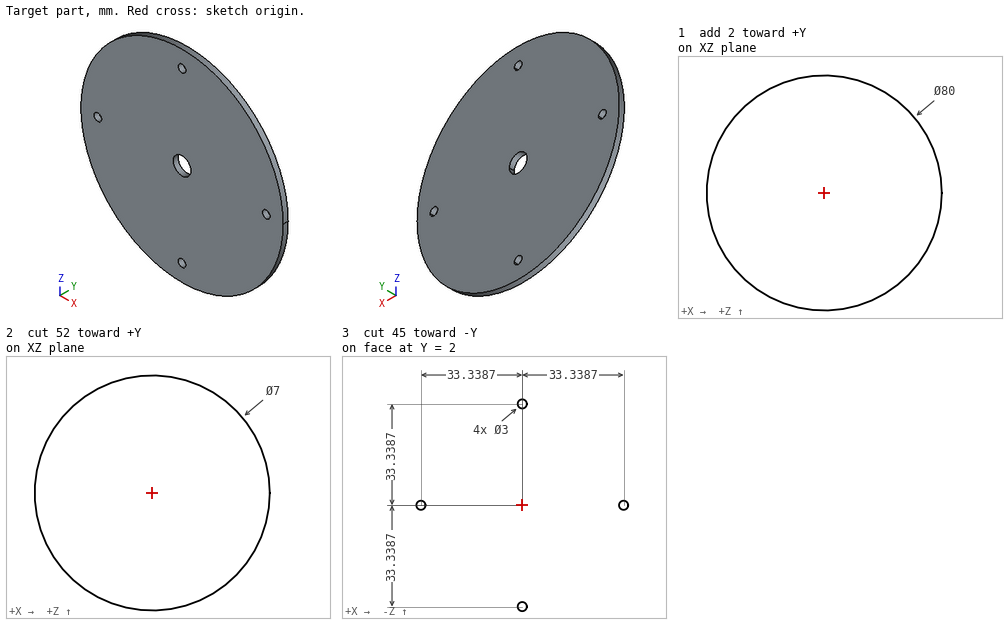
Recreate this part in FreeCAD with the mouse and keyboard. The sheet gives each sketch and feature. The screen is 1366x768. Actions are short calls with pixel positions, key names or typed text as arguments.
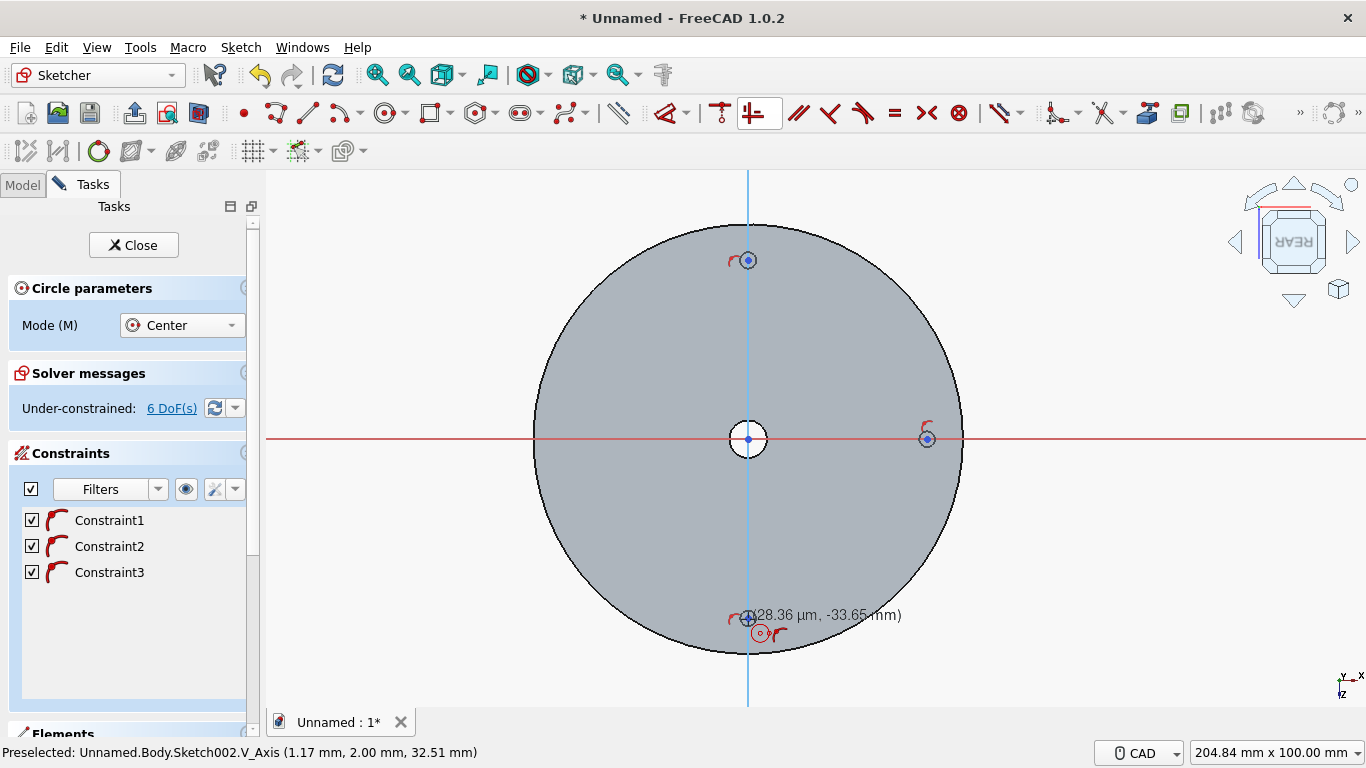
scroll(569, 439, up, 6)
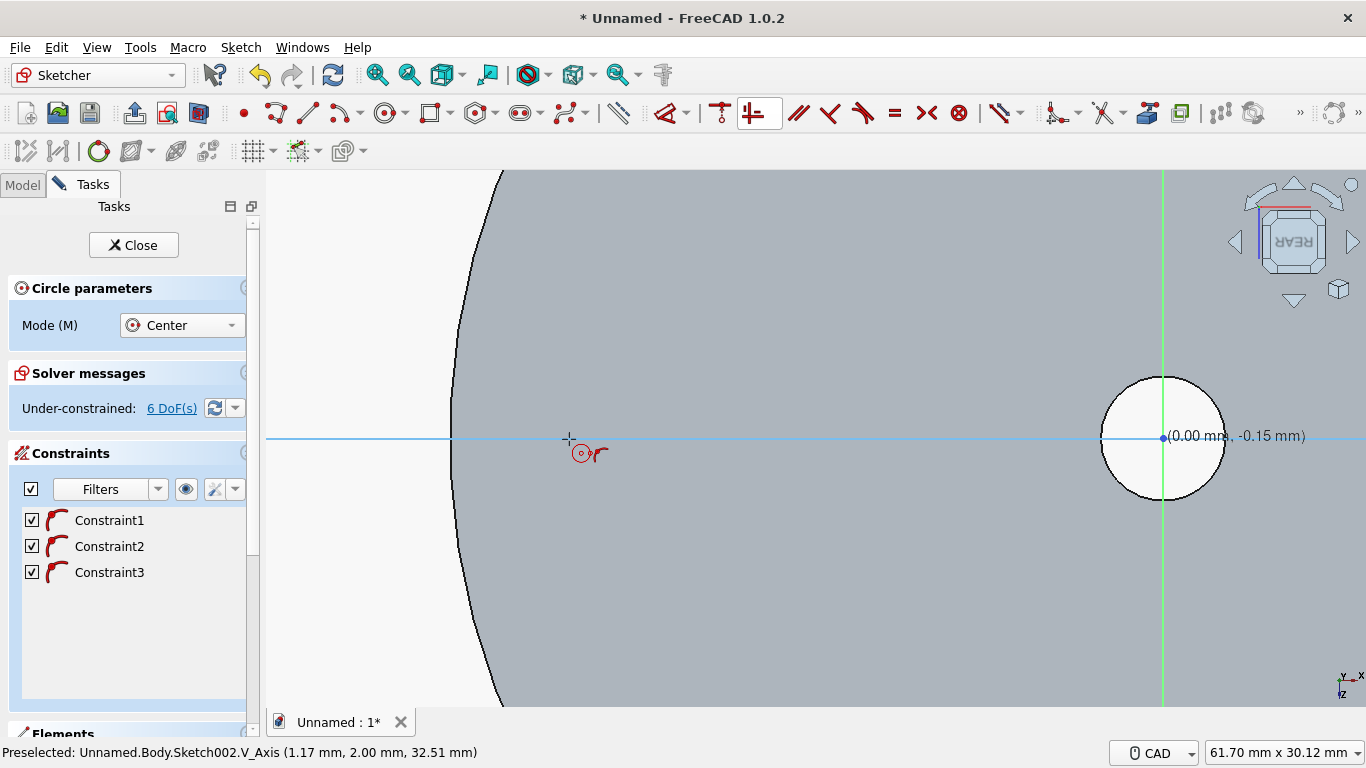
click(569, 439)
click(588, 420)
key(Escape)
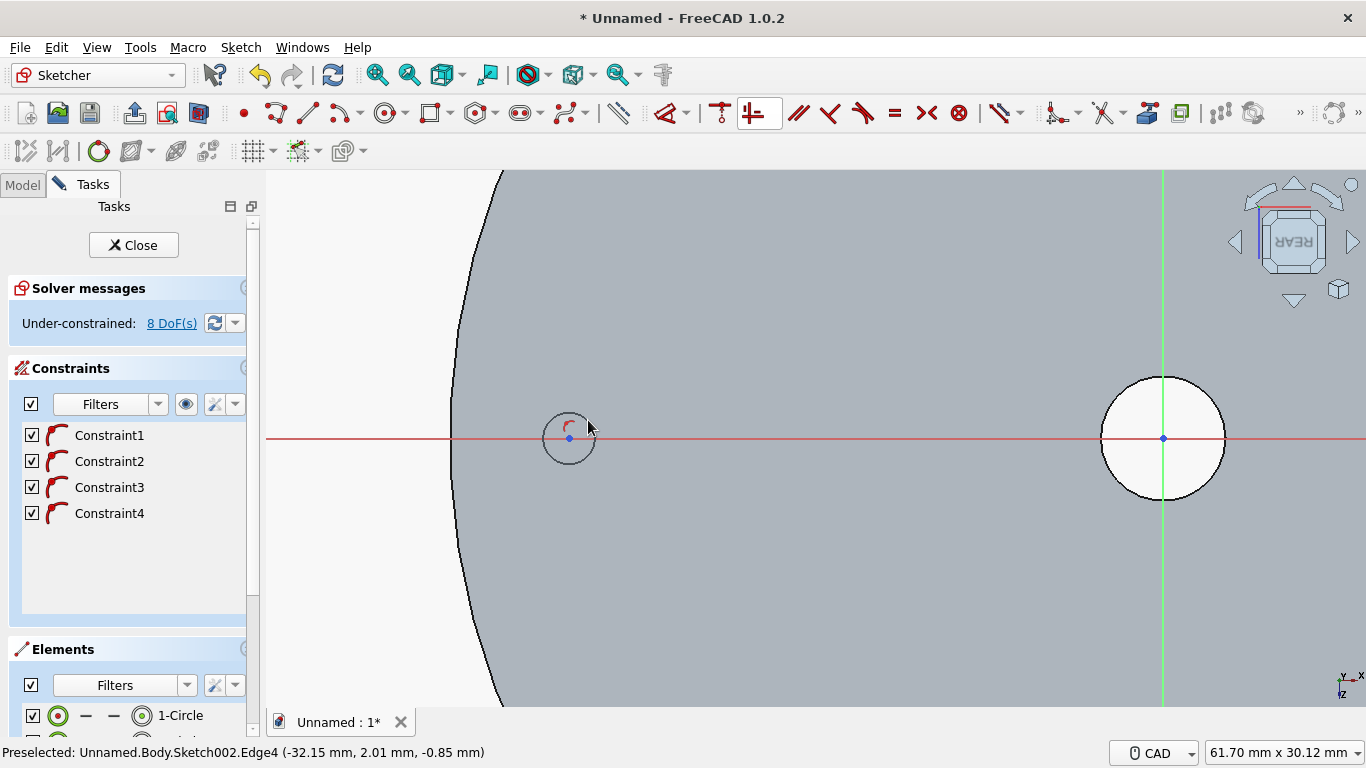
scroll(568, 438, down, 6)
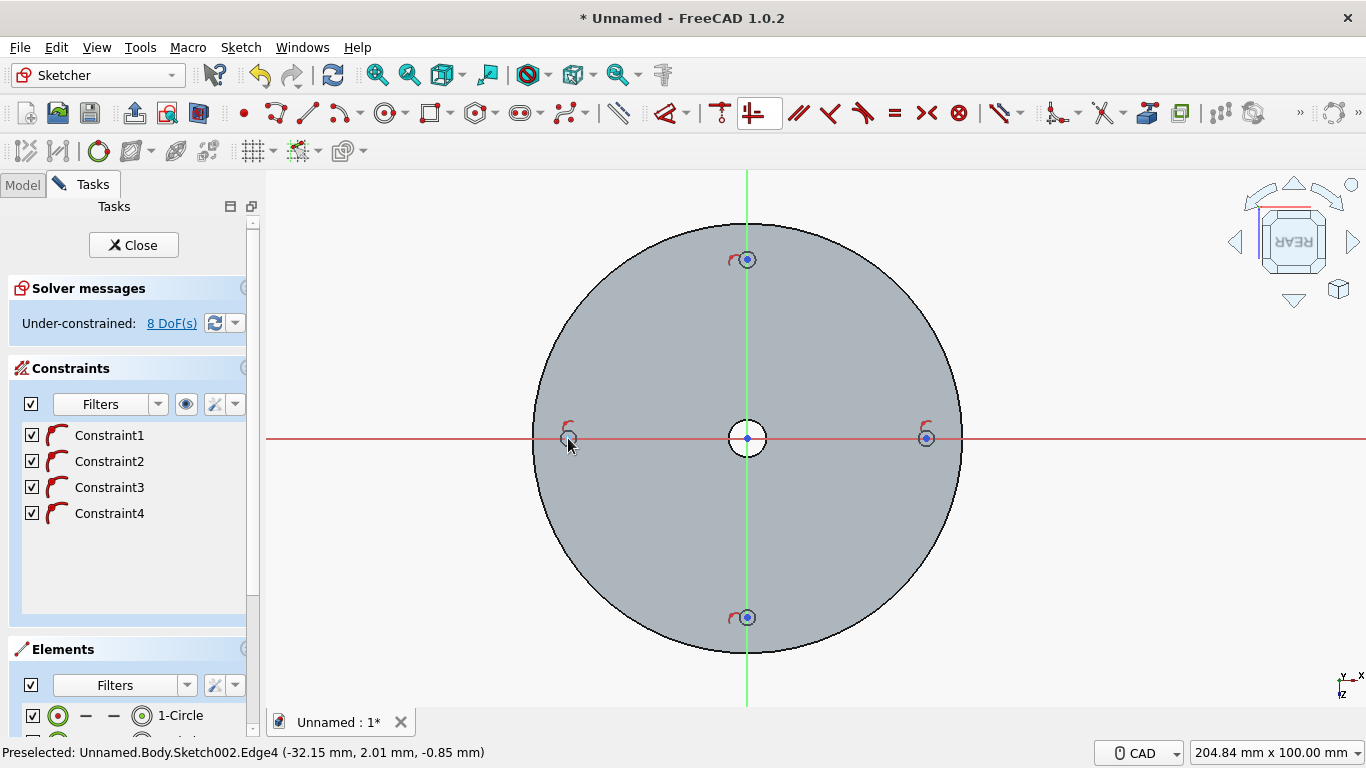
scroll(753, 254, up, 5)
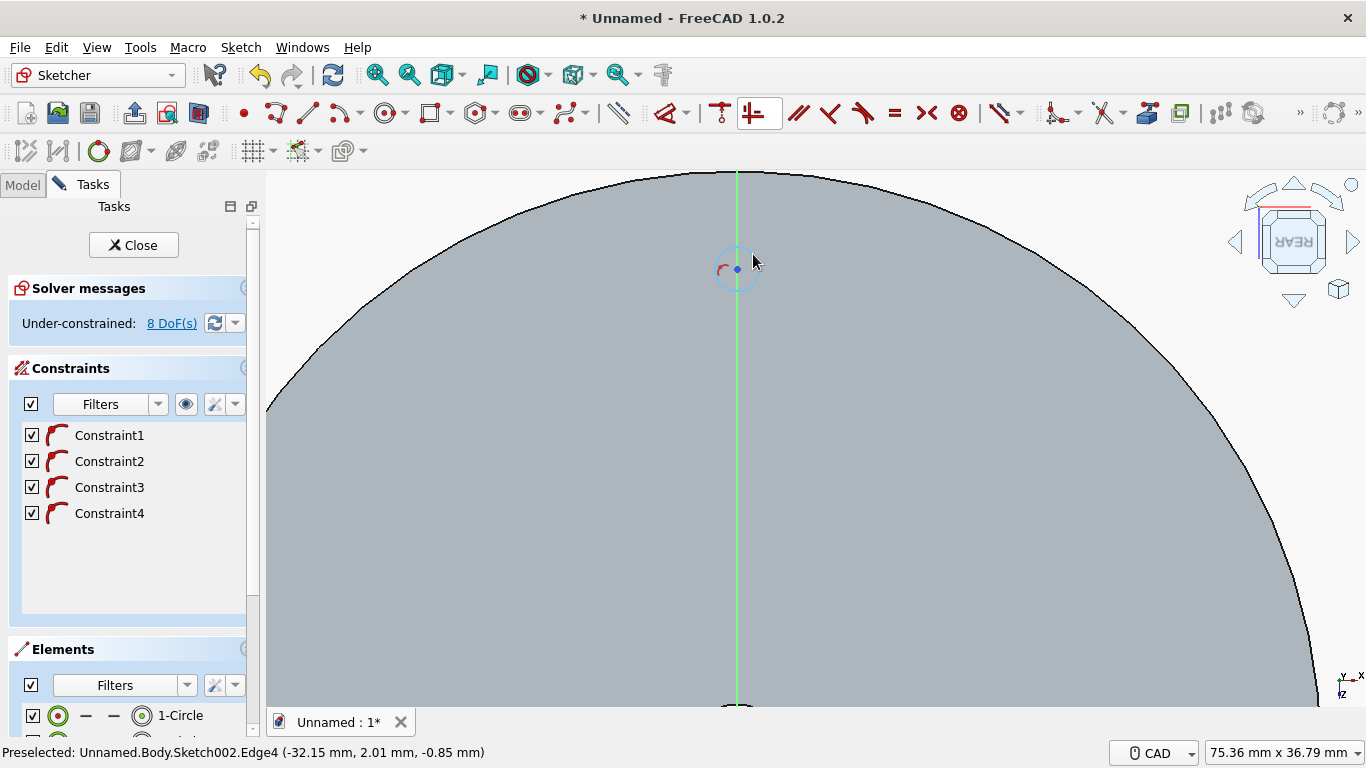
click(753, 254)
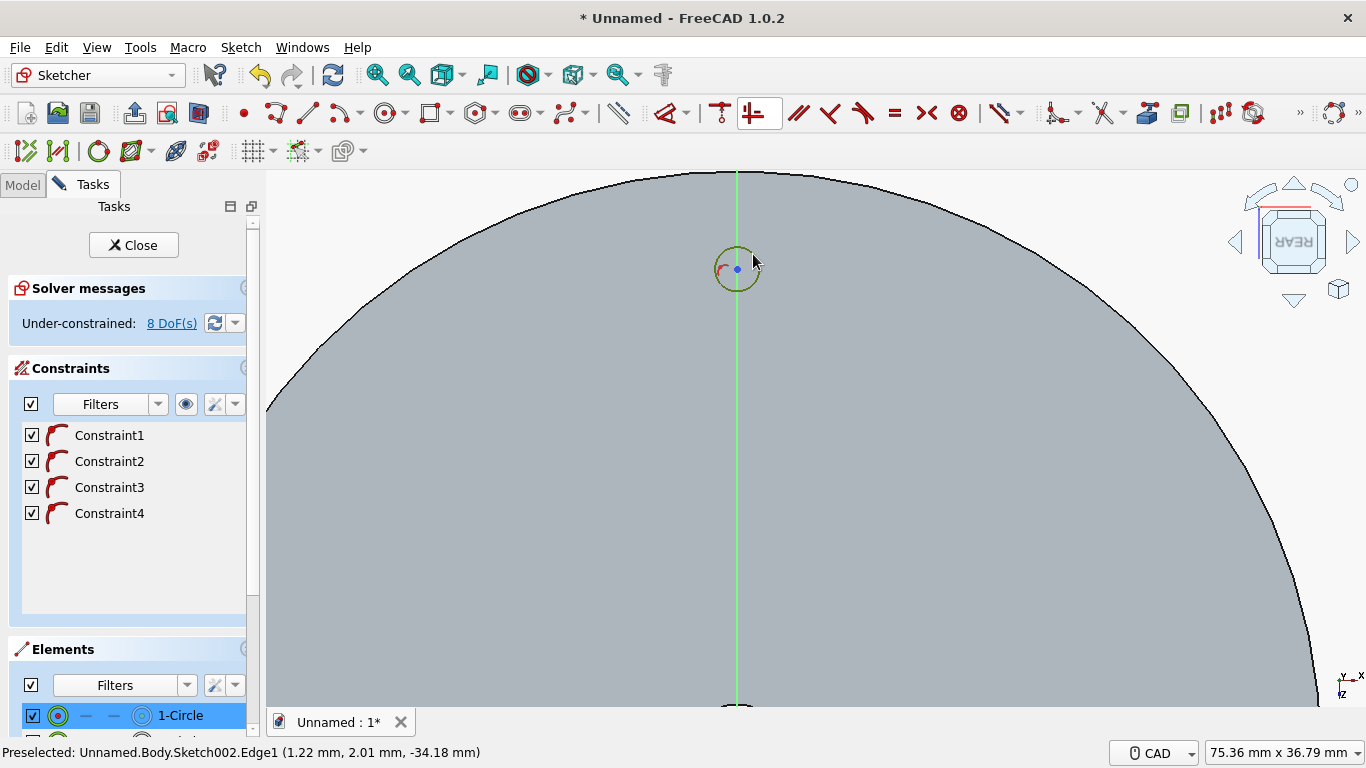
scroll(754, 254, down, 5)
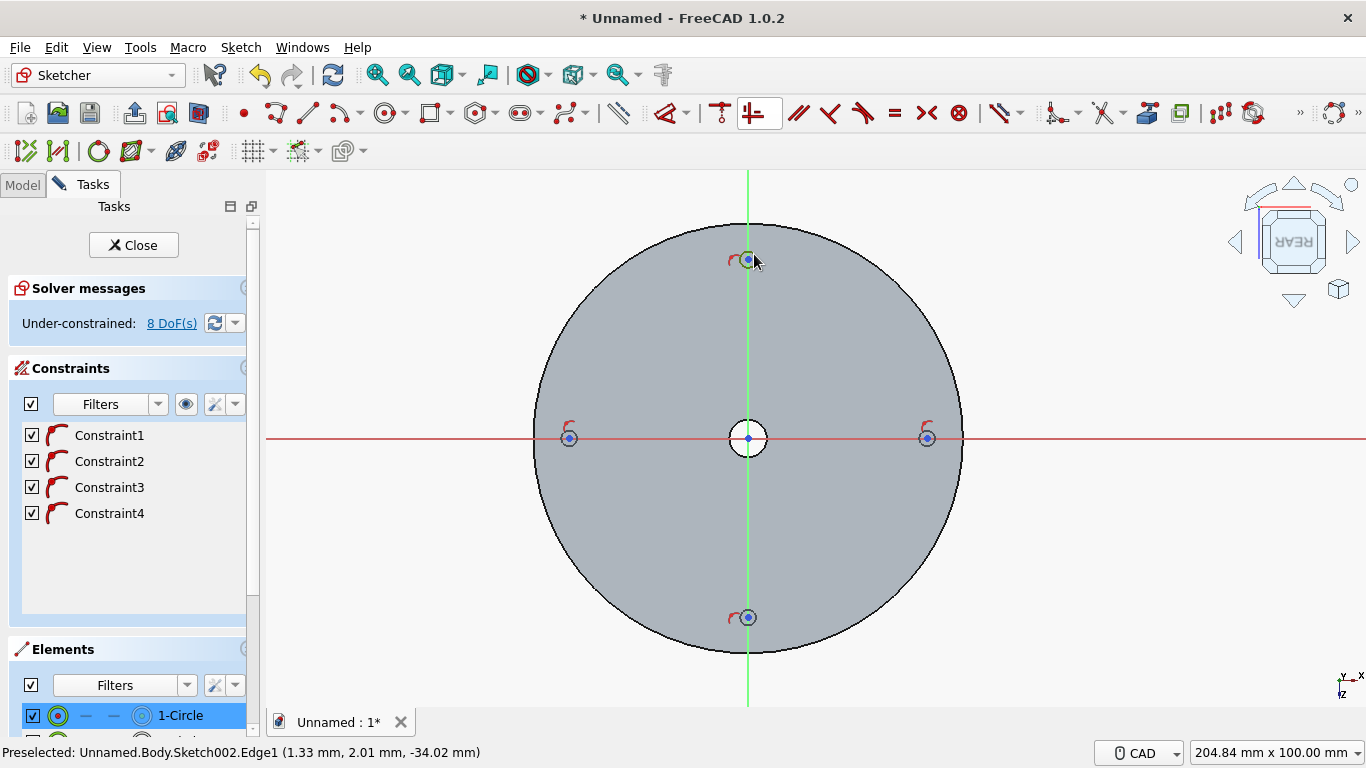
scroll(933, 433, up, 5)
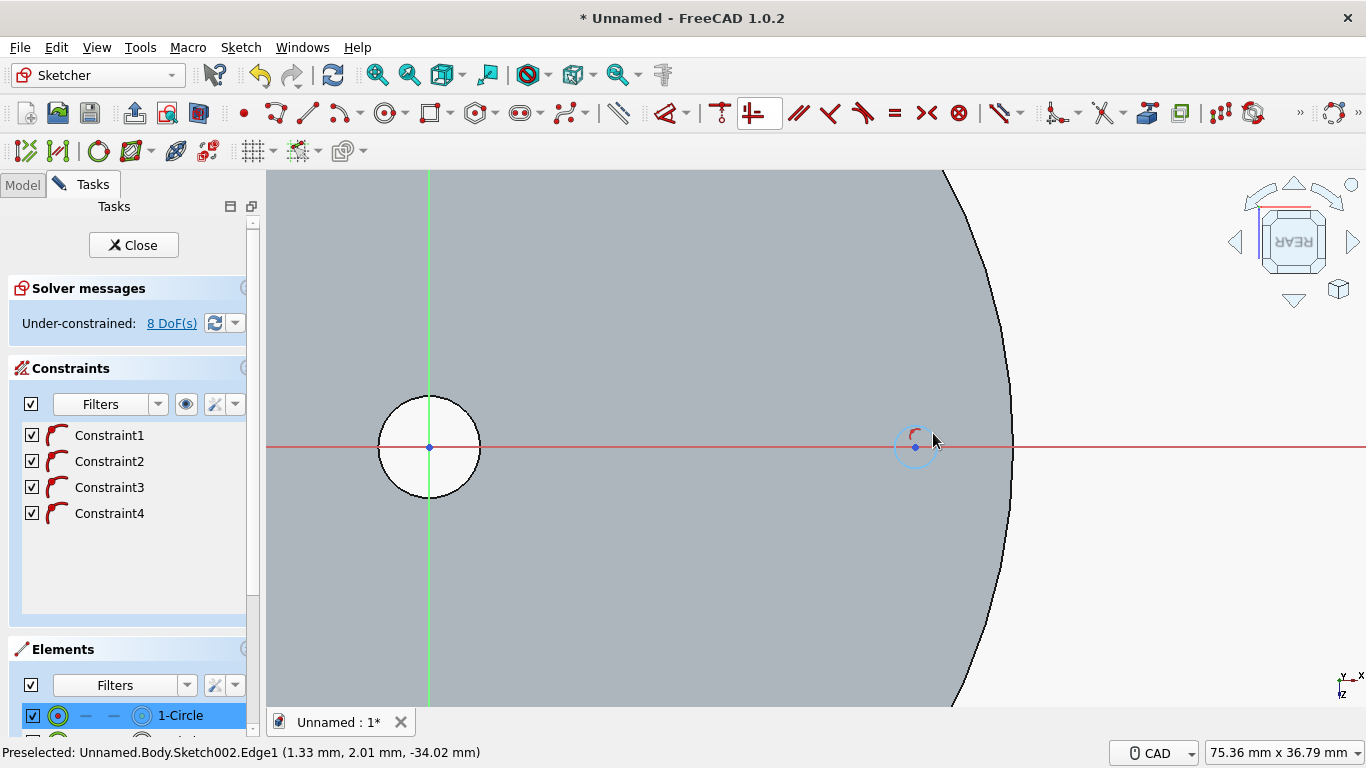
click(931, 432)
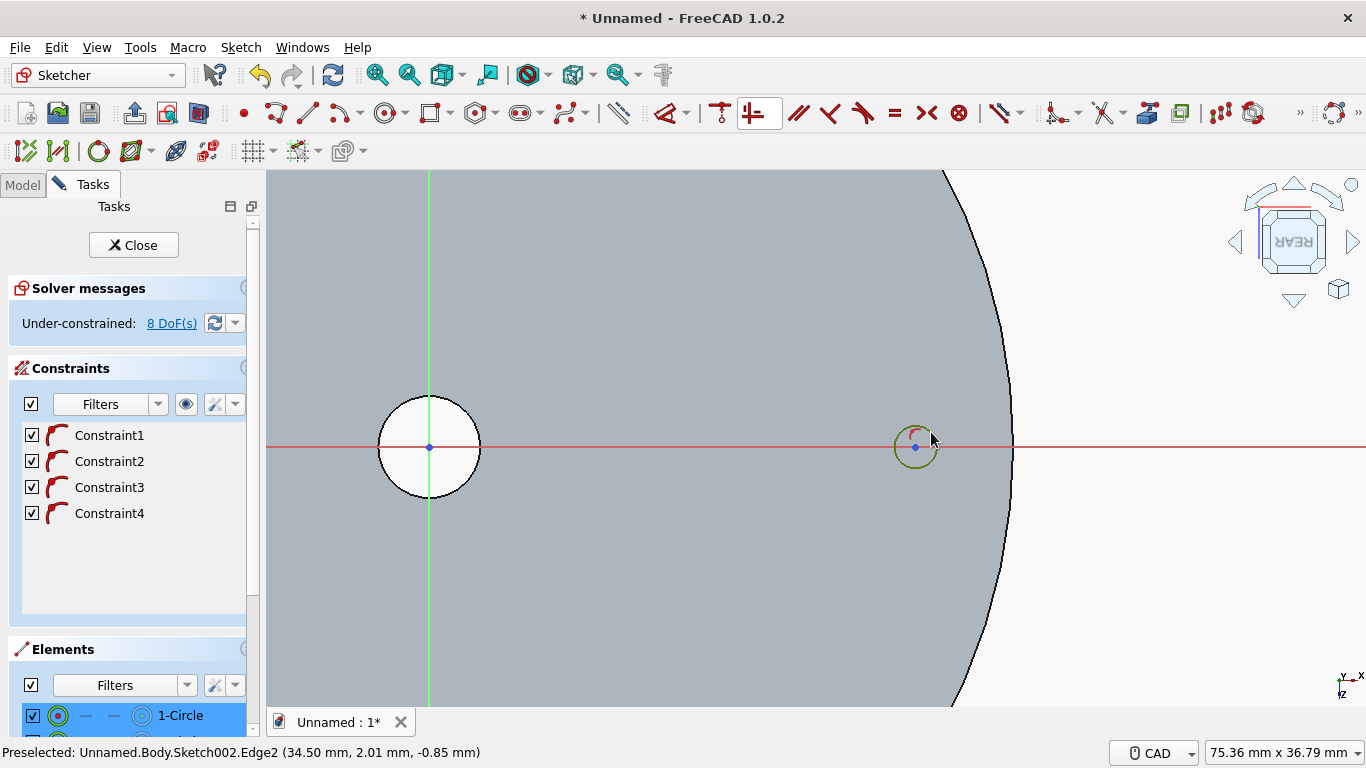
scroll(933, 433, down, 5)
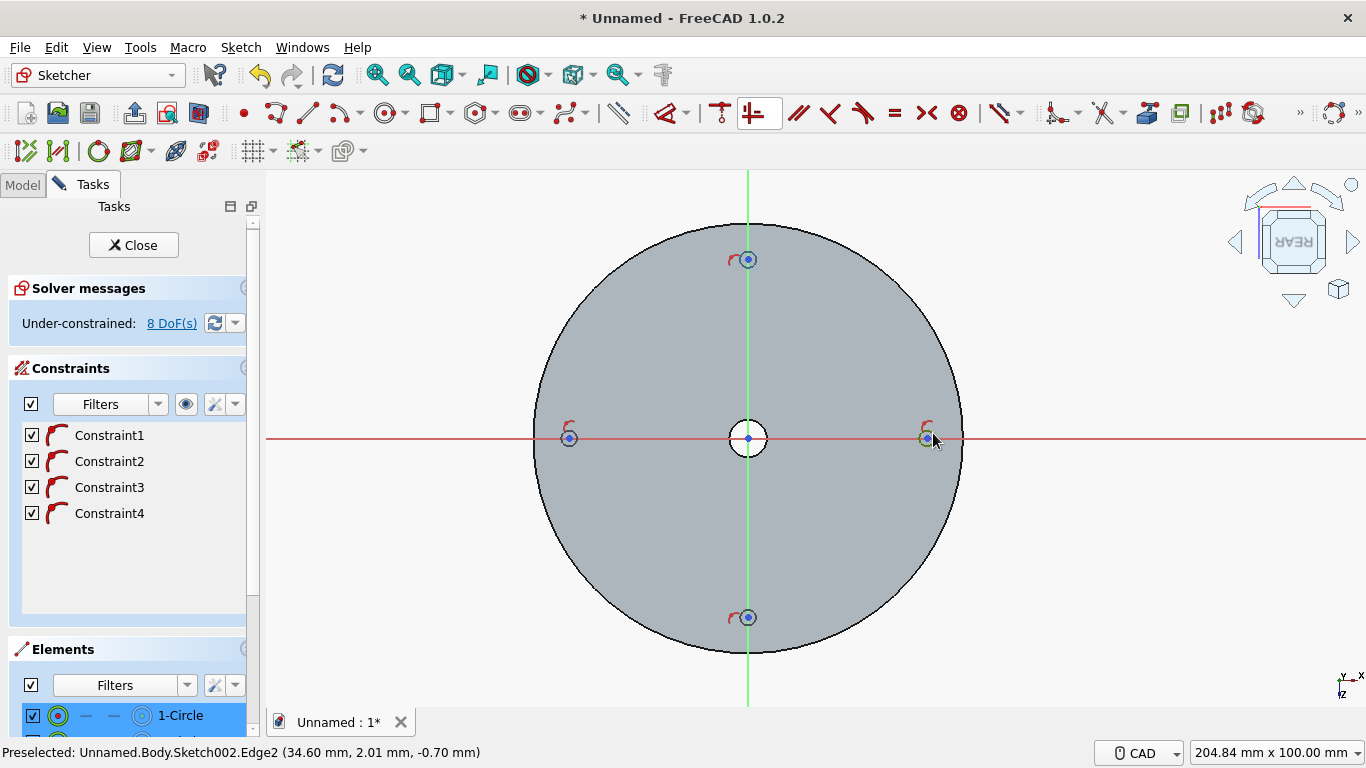
scroll(754, 612, up, 5)